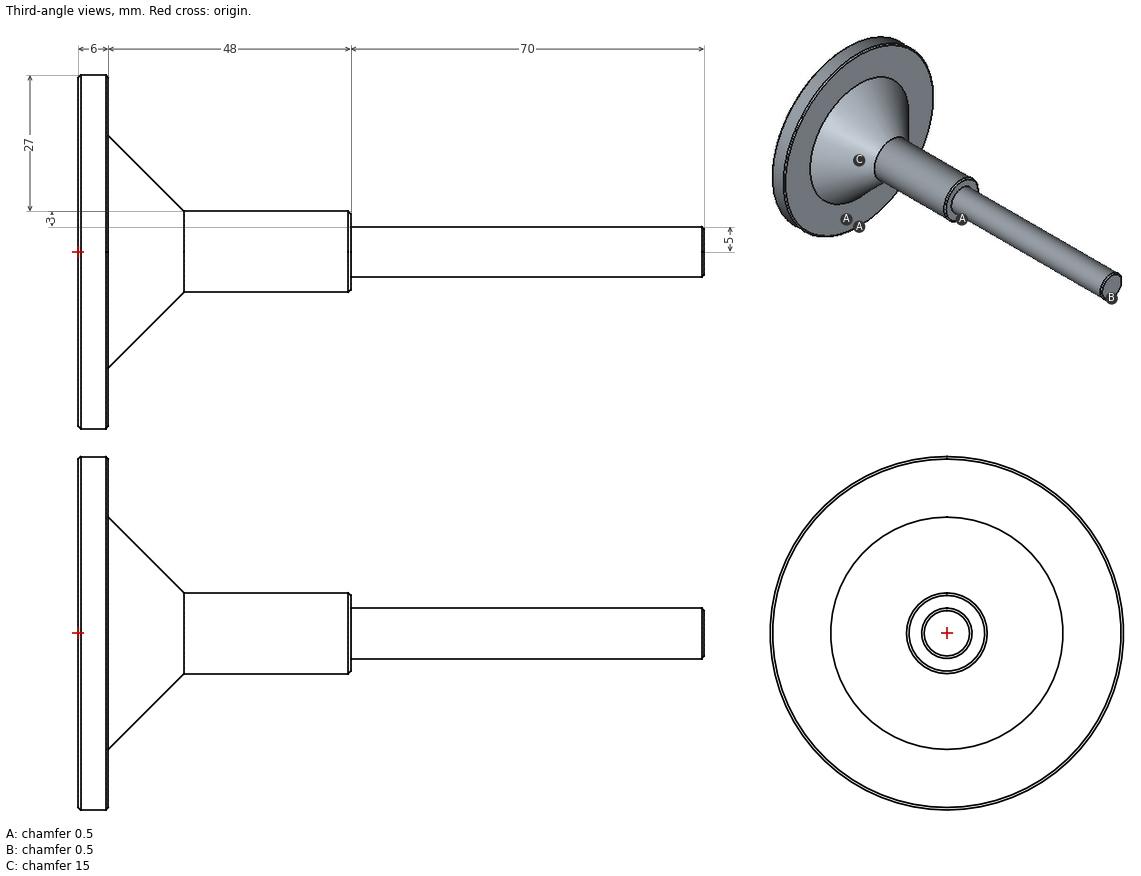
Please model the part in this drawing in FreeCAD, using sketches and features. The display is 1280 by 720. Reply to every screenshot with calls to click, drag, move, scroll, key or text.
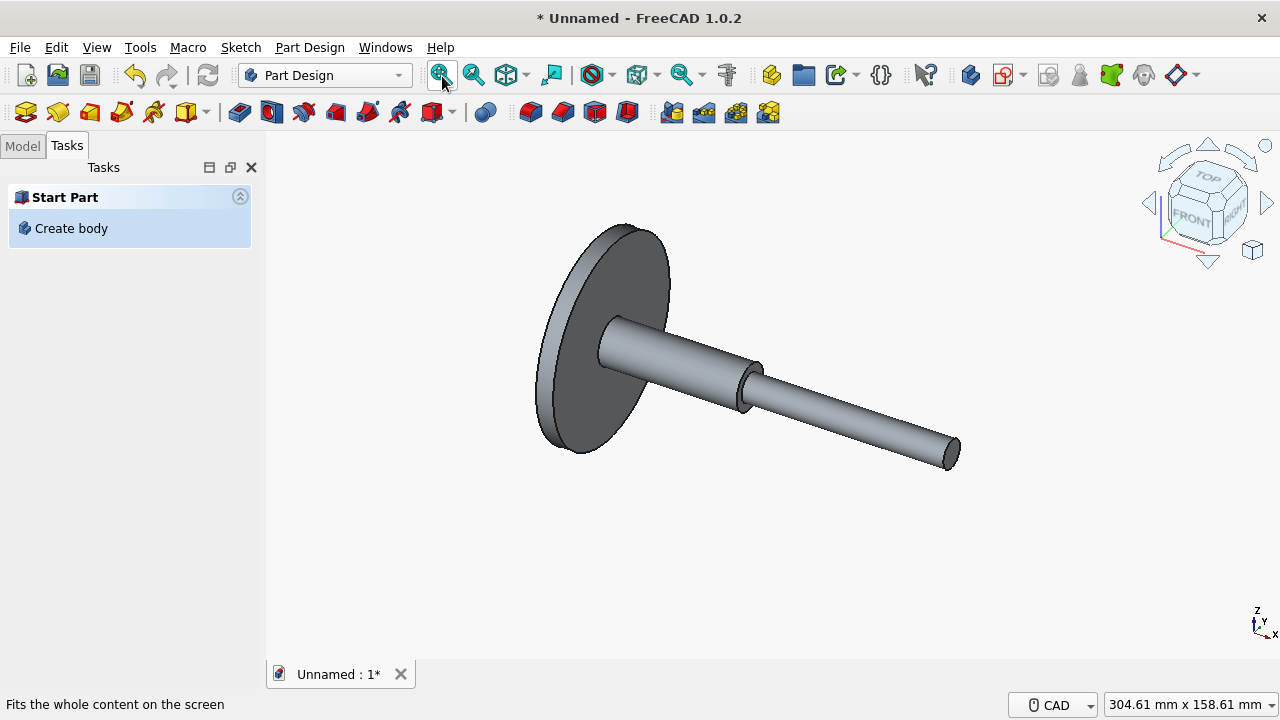
click(737, 400)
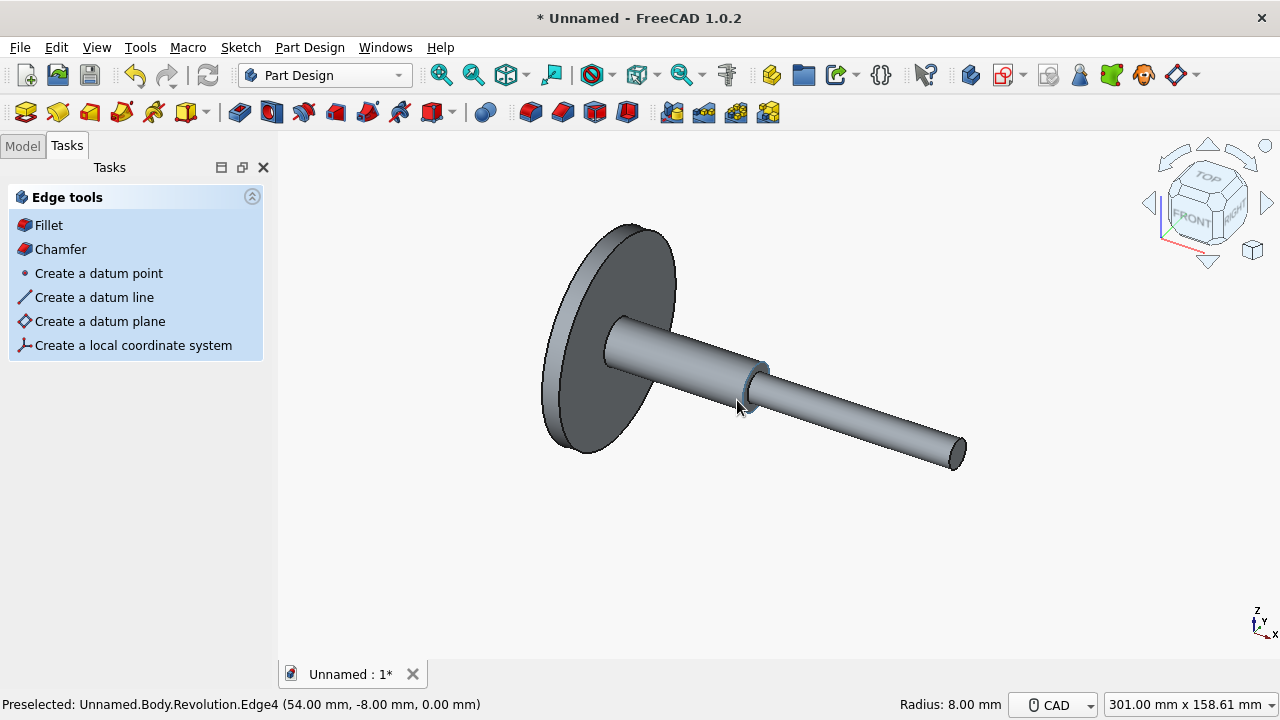
click(559, 398, ctrl)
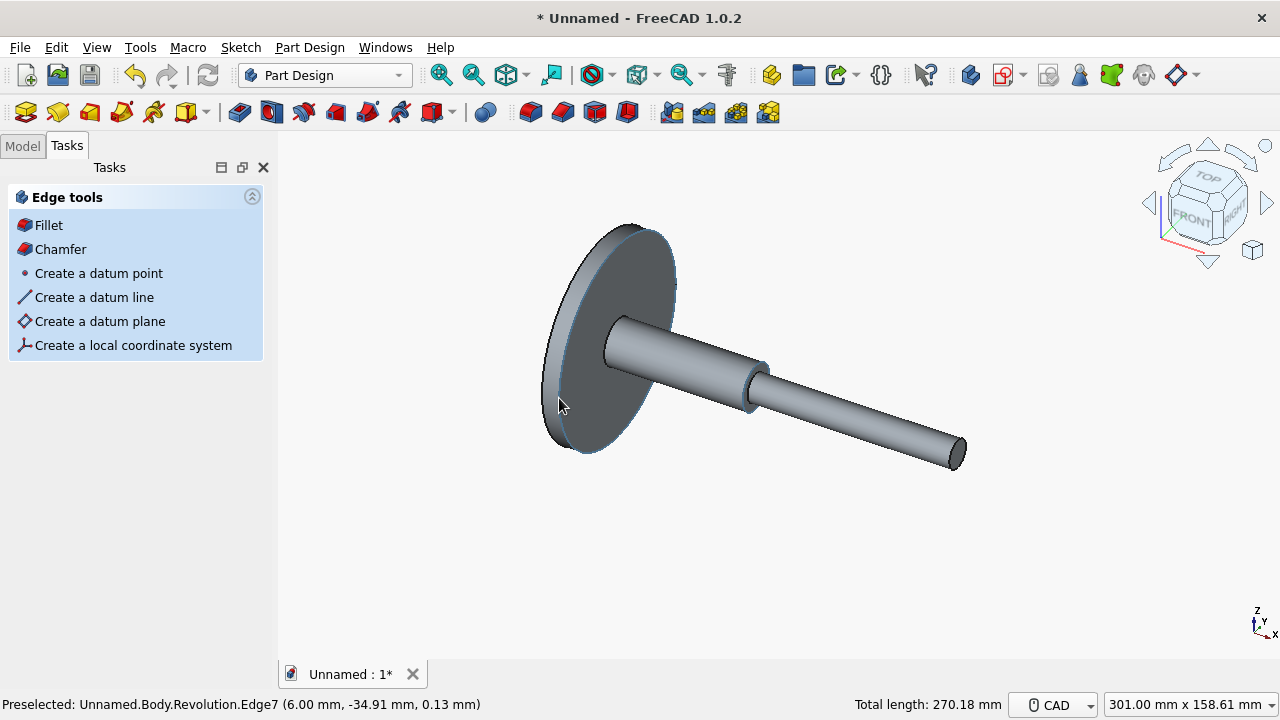
key(0)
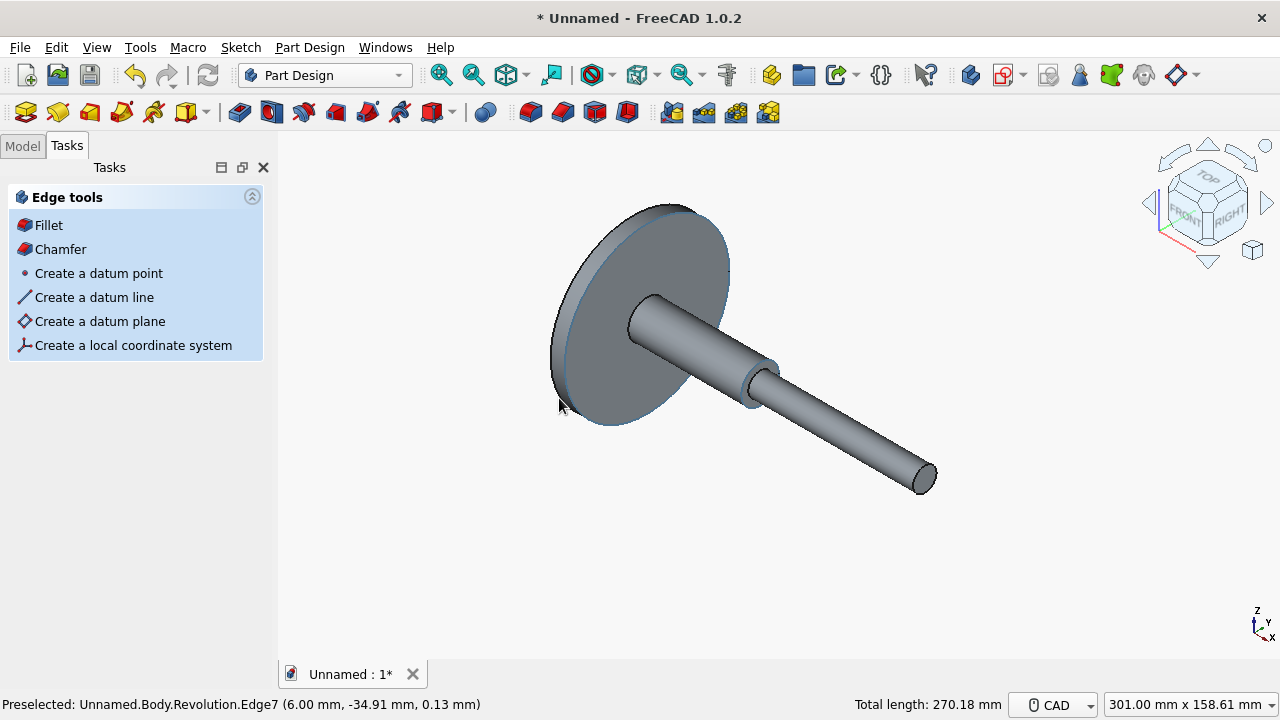
key(2)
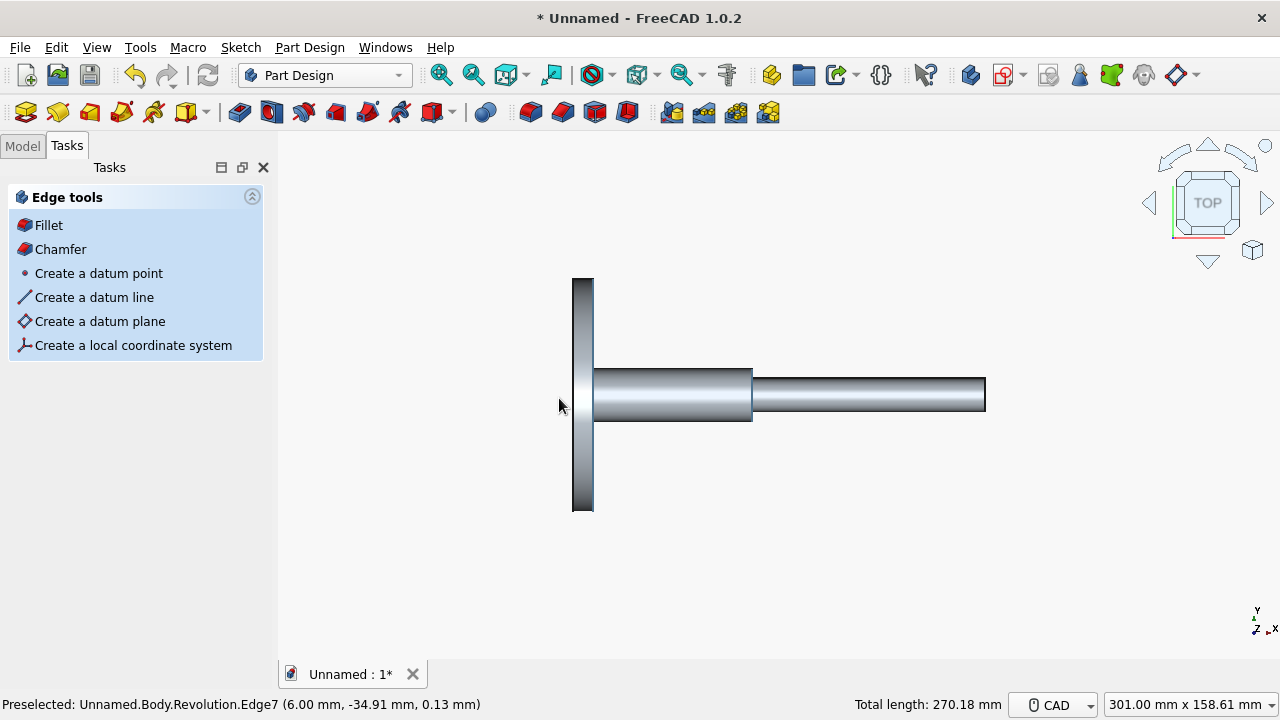
click(442, 76)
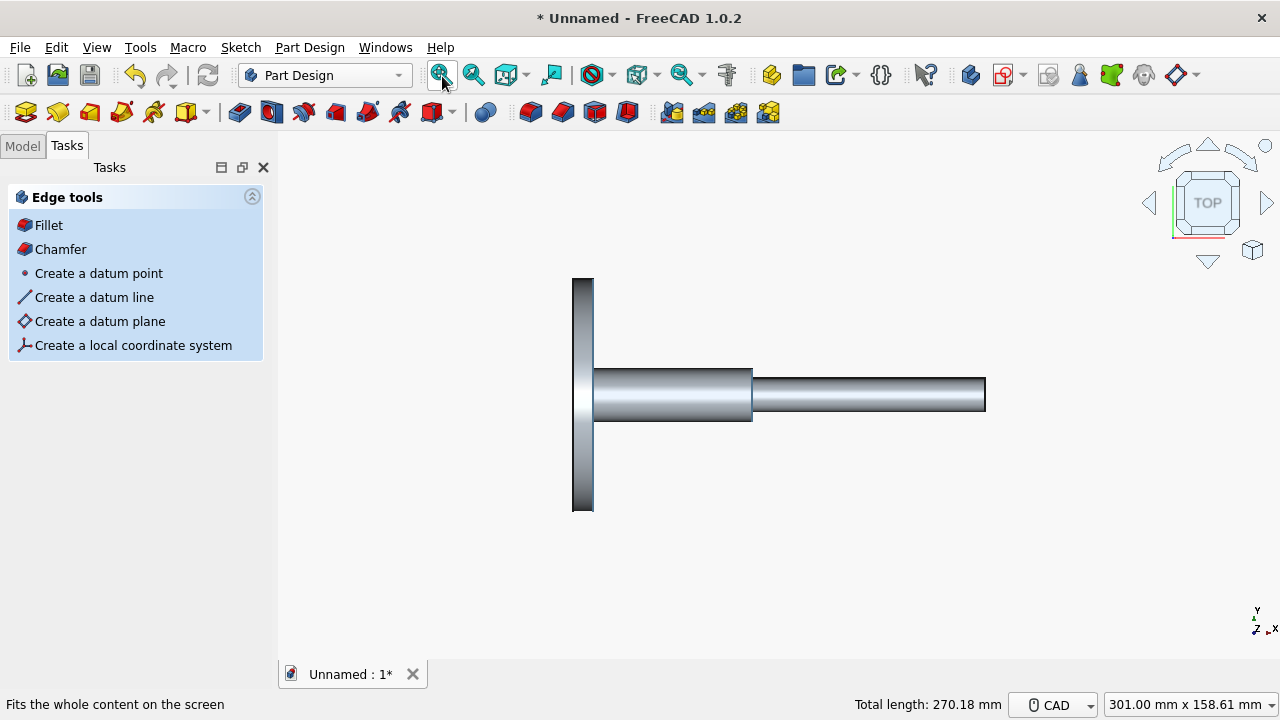
click(573, 488, ctrl)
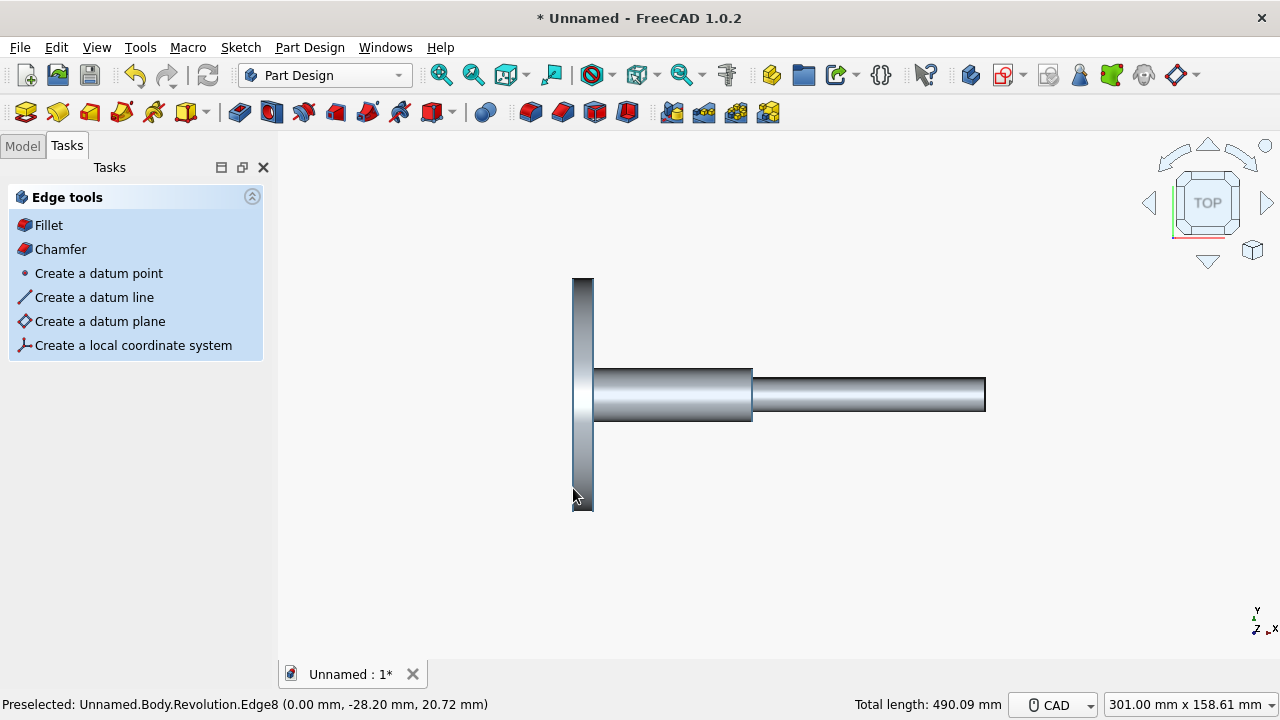
click(564, 112)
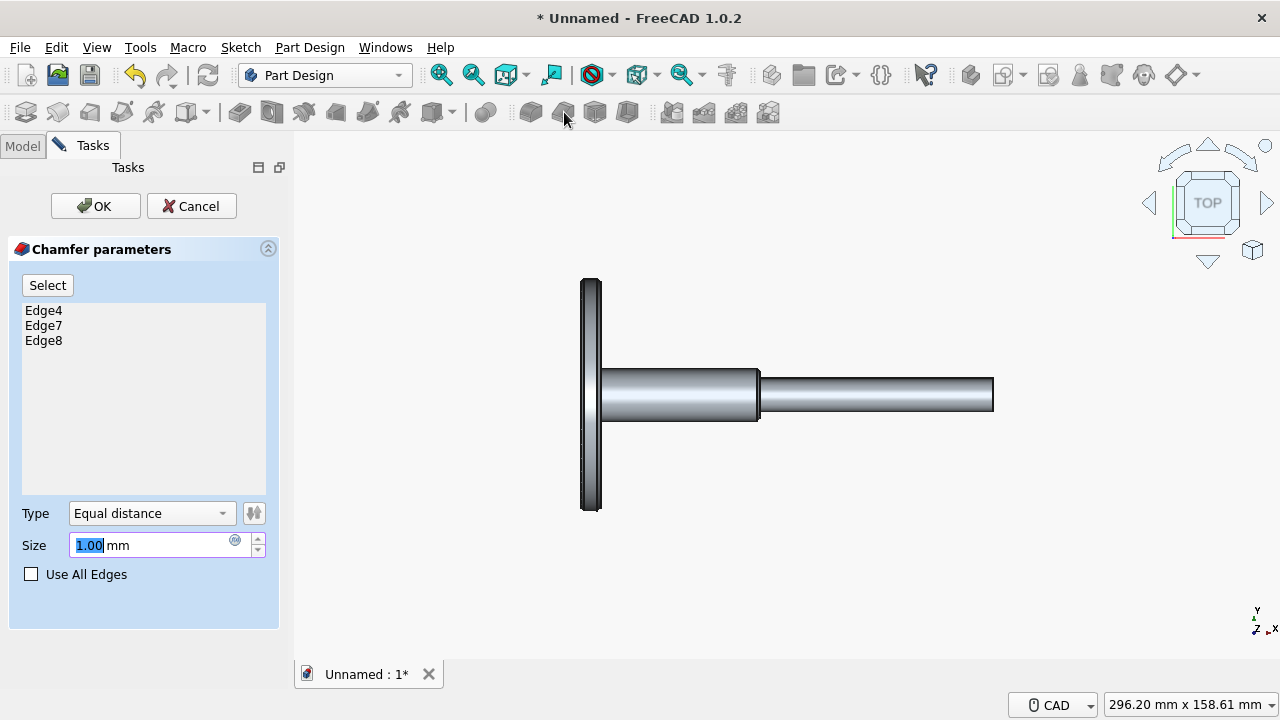
text(0.5)
key(Tab)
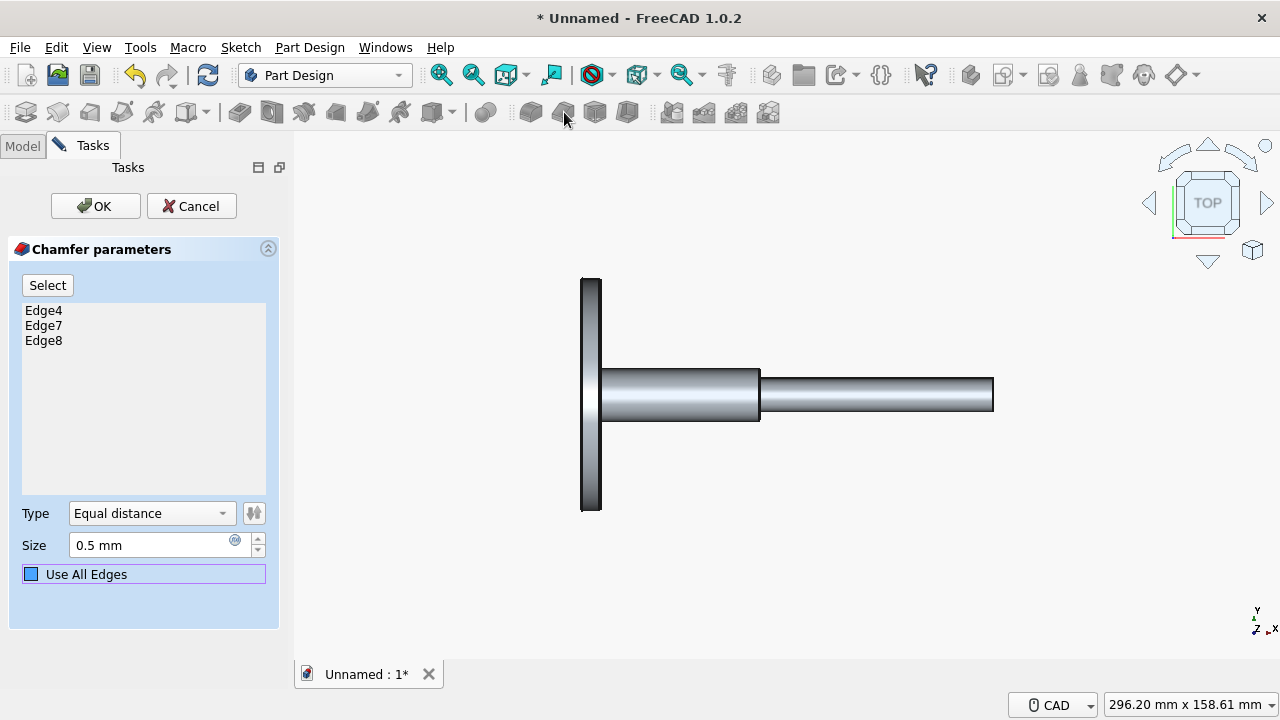
click(96, 206)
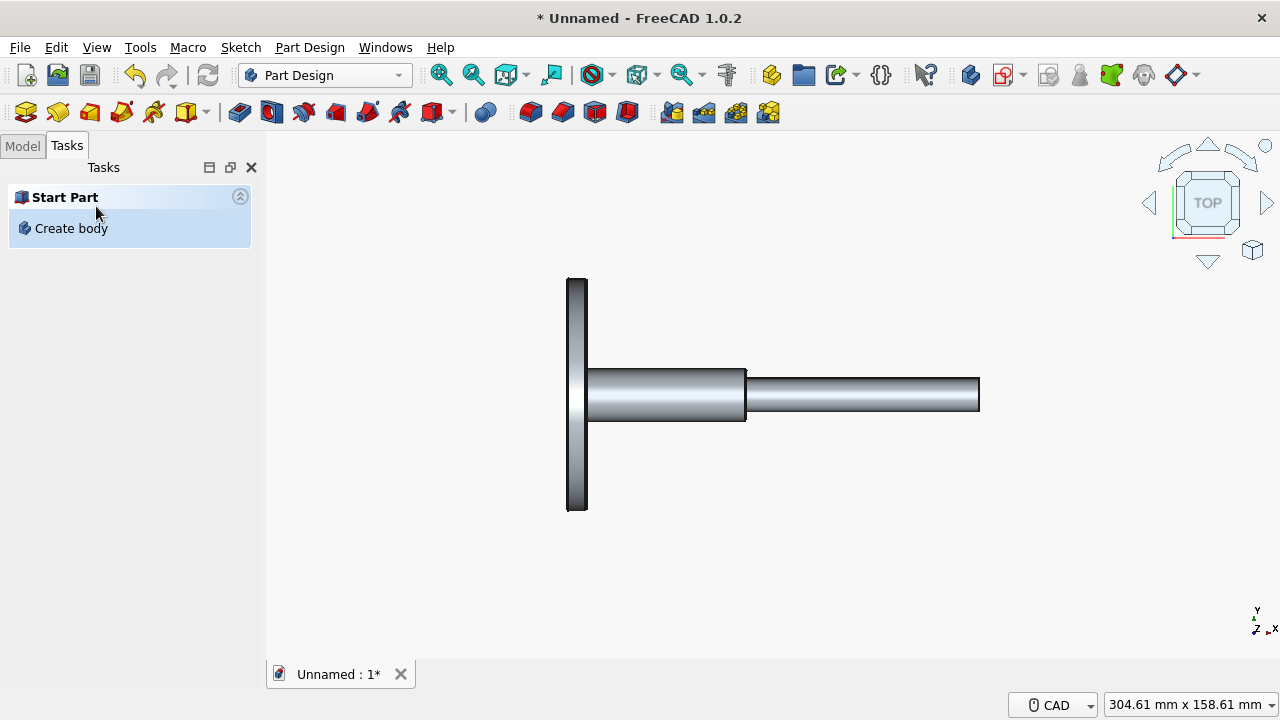
click(442, 76)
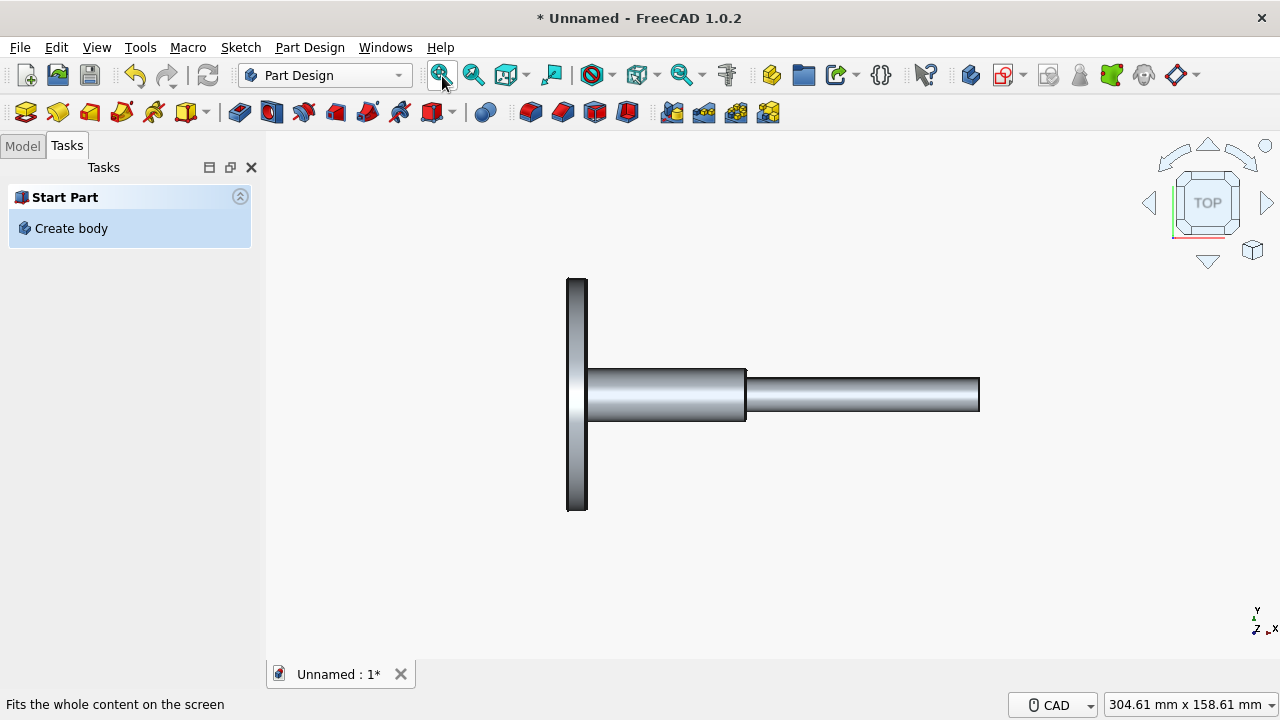
click(979, 411)